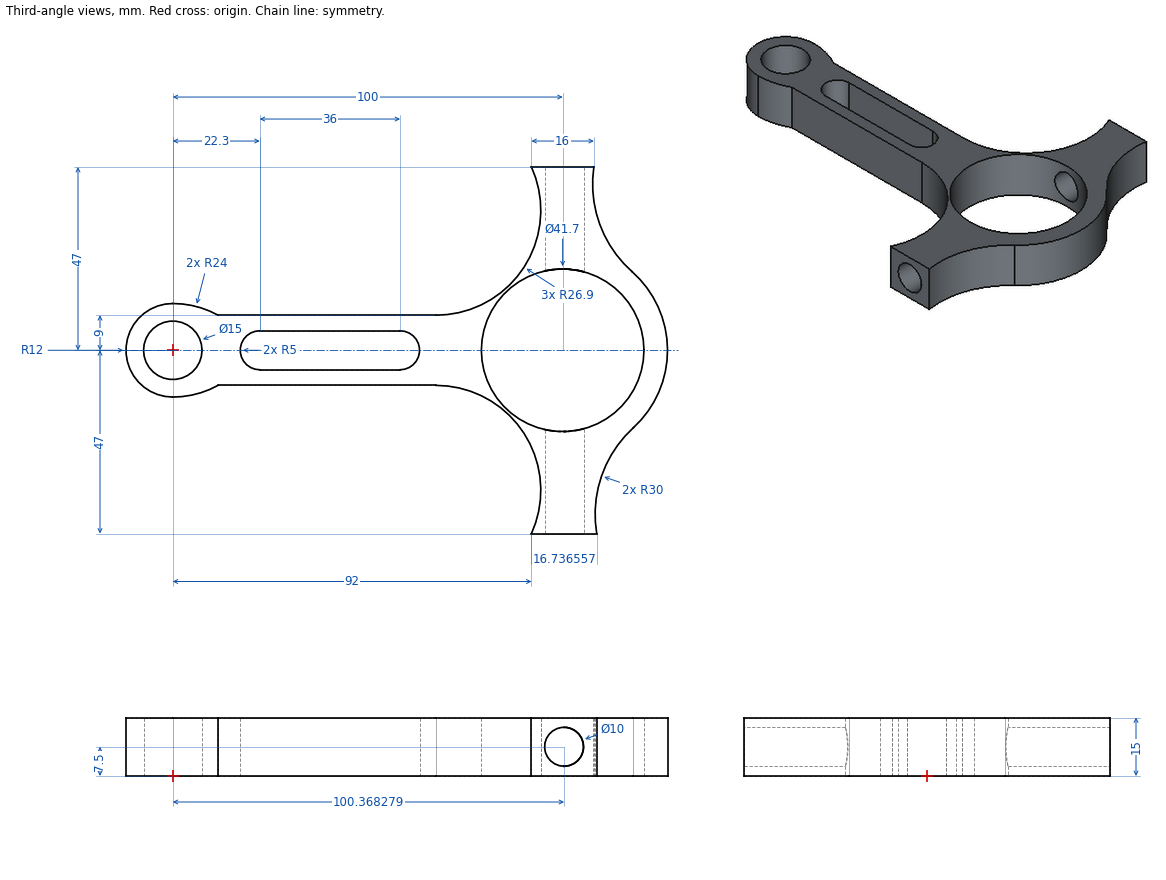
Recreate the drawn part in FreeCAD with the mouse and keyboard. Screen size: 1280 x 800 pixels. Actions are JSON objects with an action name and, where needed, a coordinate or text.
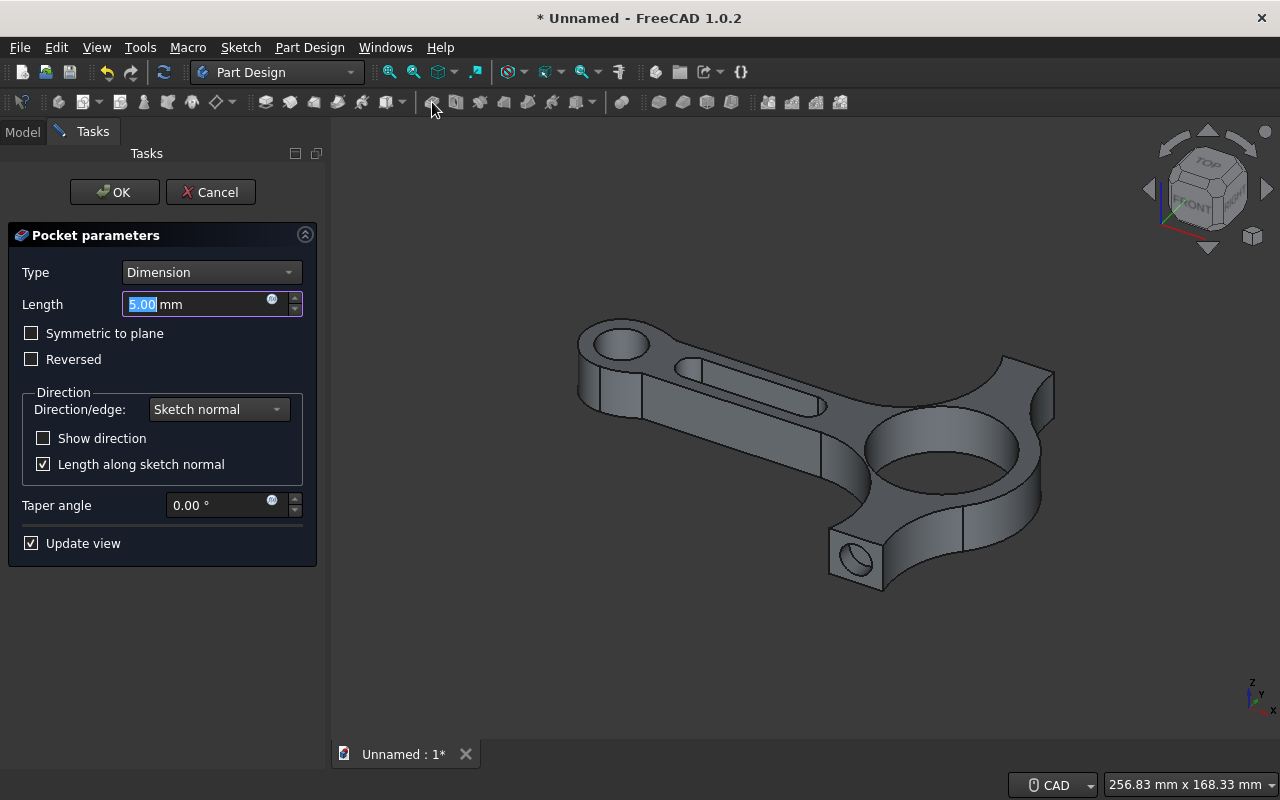
{"action": "left_click", "coordinate": [212, 272]}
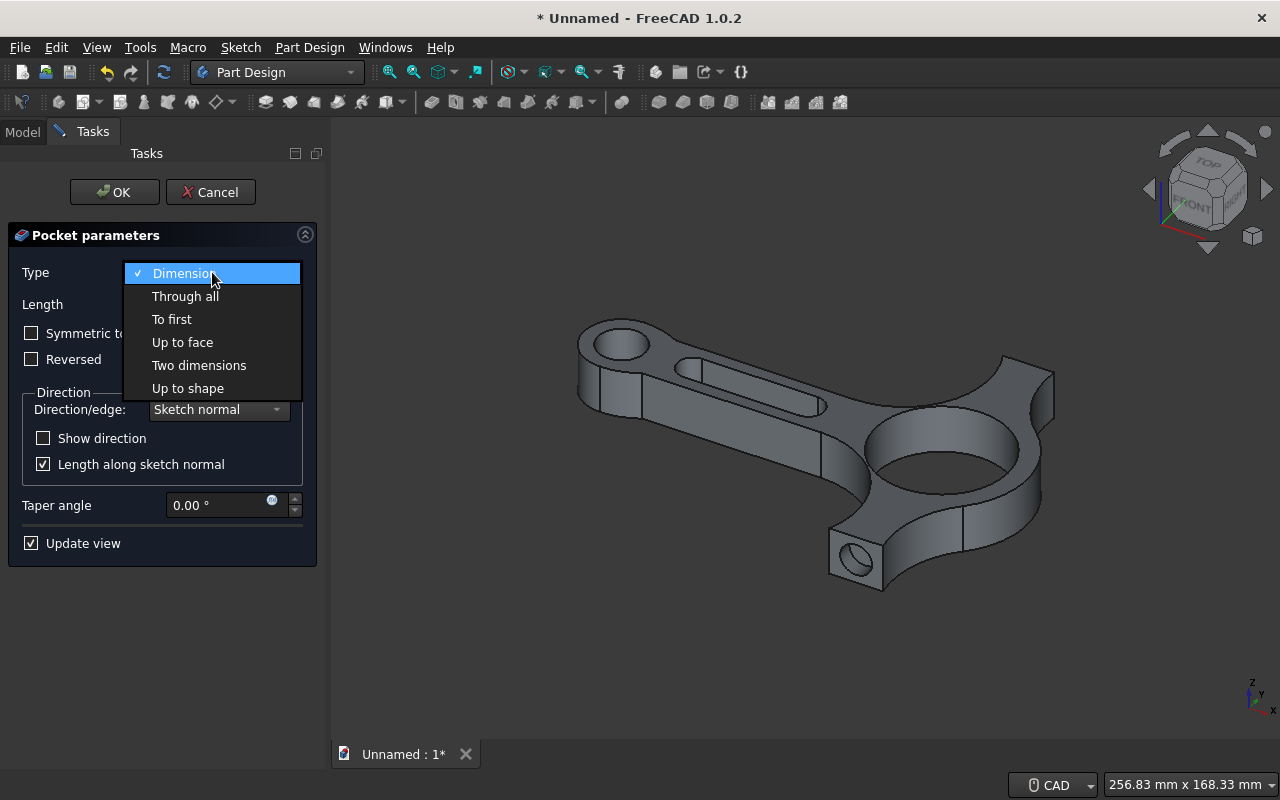
{"action": "left_click", "coordinate": [212, 296]}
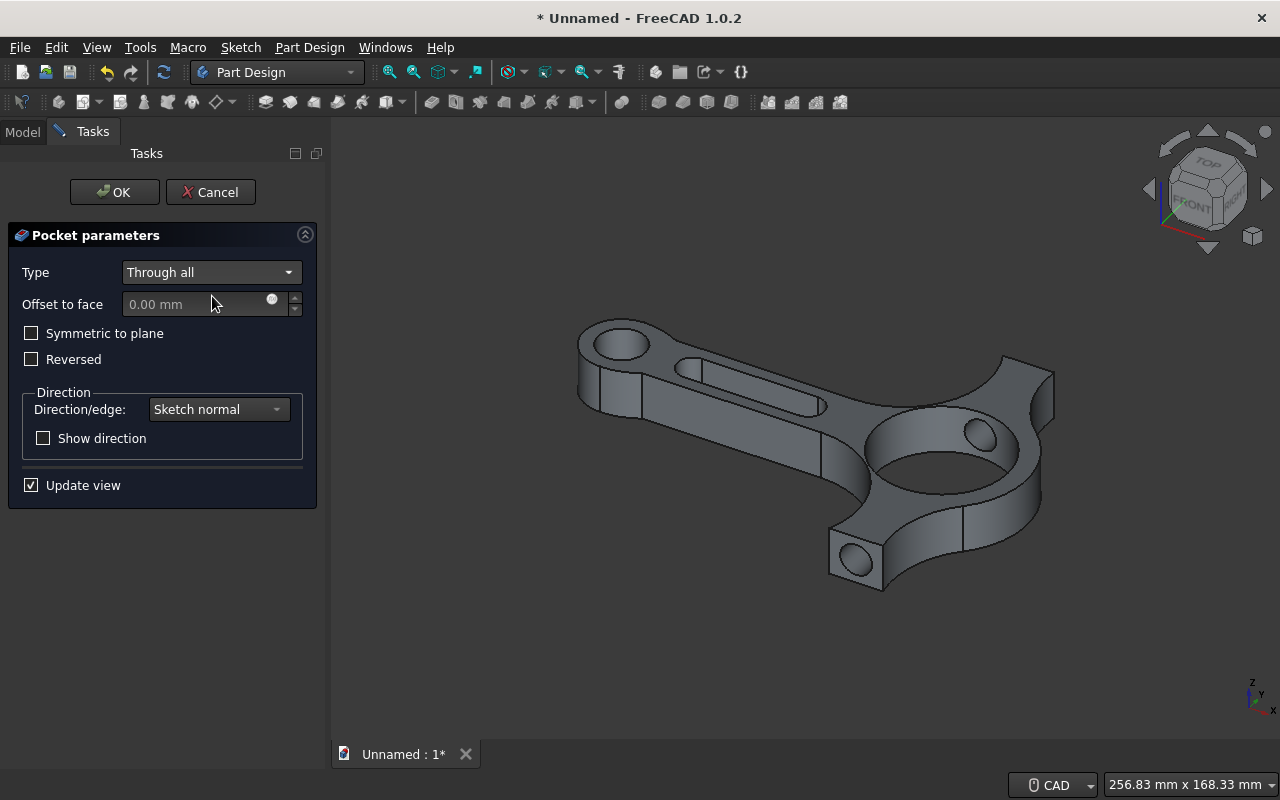
{"action": "left_click", "coordinate": [115, 192]}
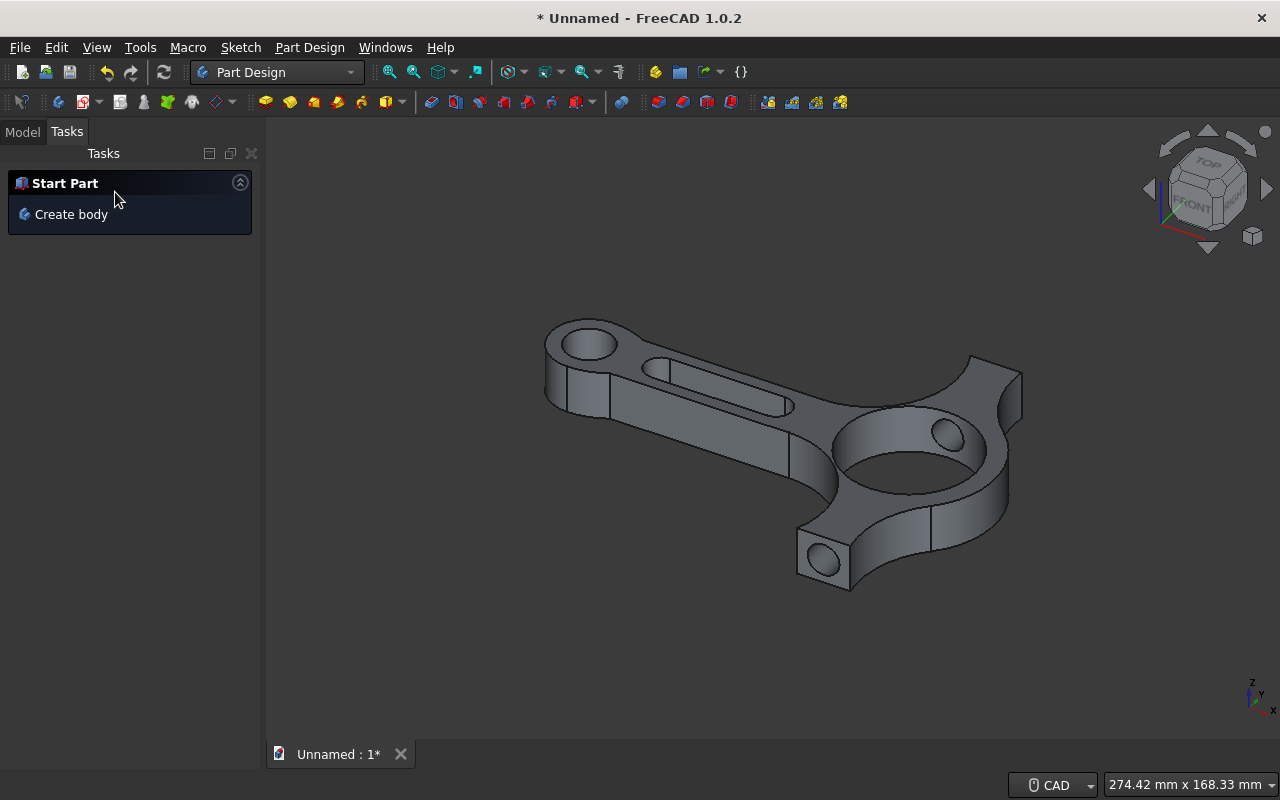
{"action": "key", "text": "0"}